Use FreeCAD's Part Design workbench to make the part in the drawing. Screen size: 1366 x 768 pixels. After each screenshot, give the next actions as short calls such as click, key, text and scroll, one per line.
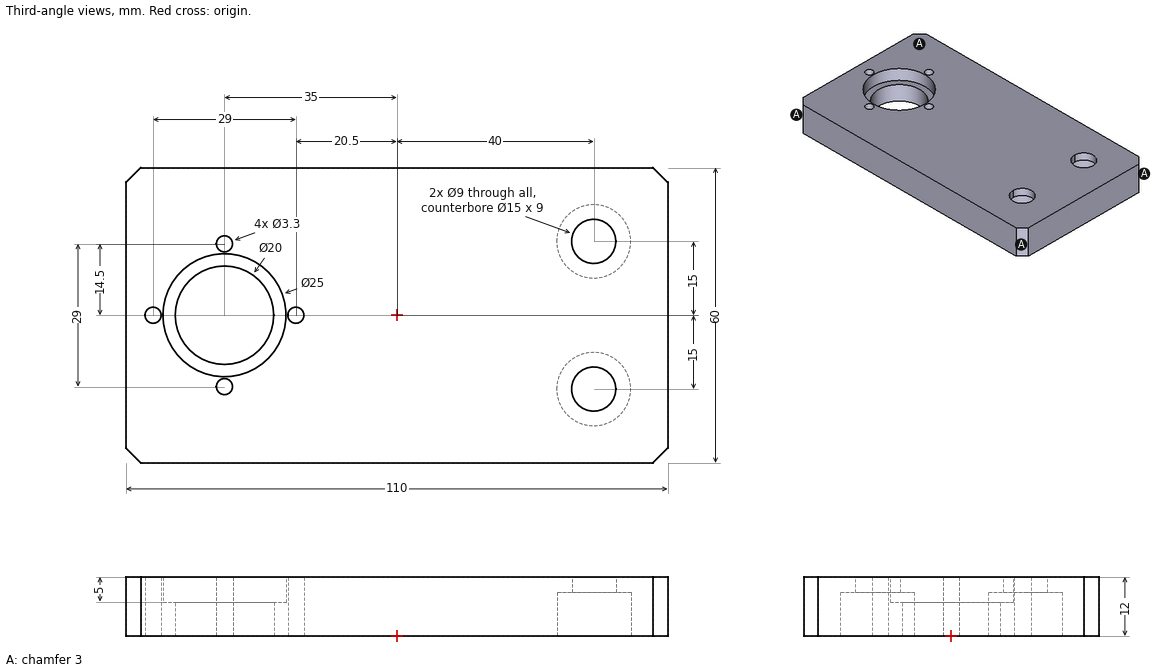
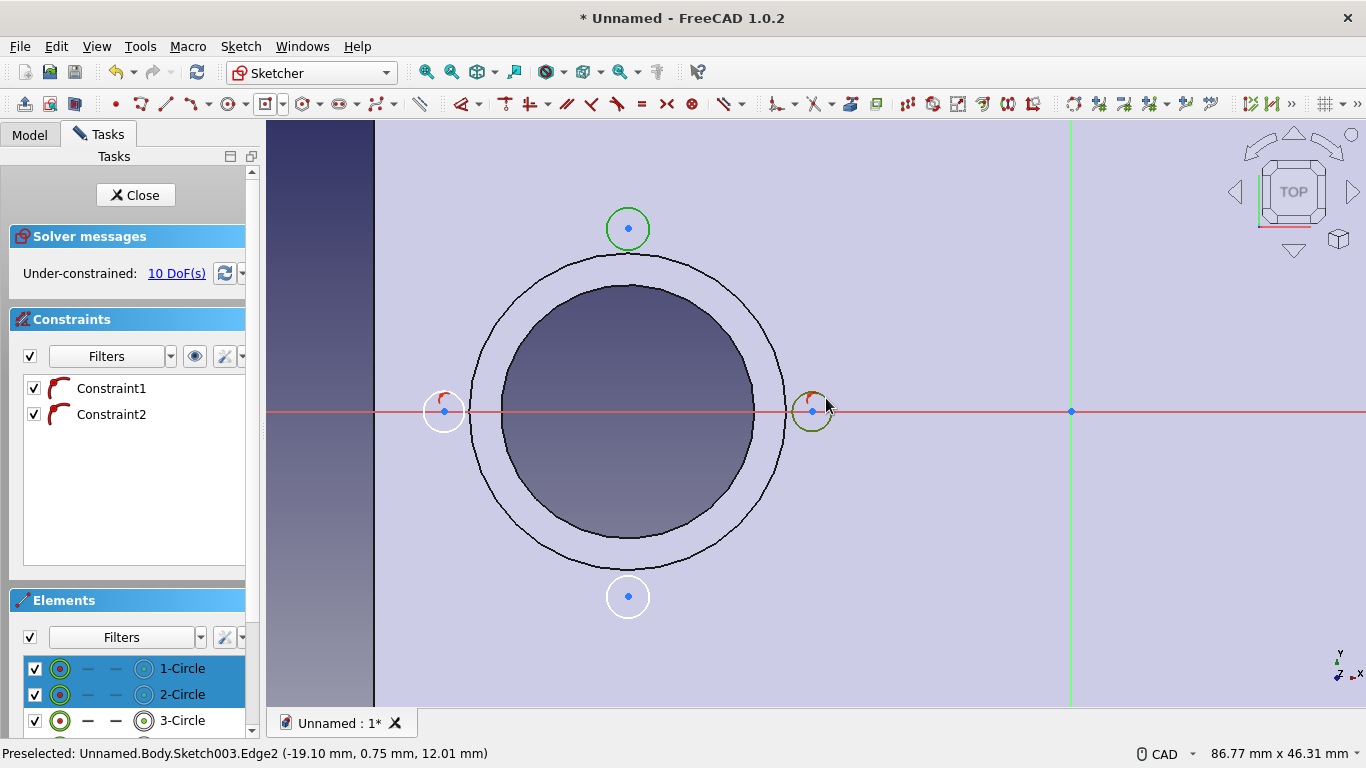
click(458, 397)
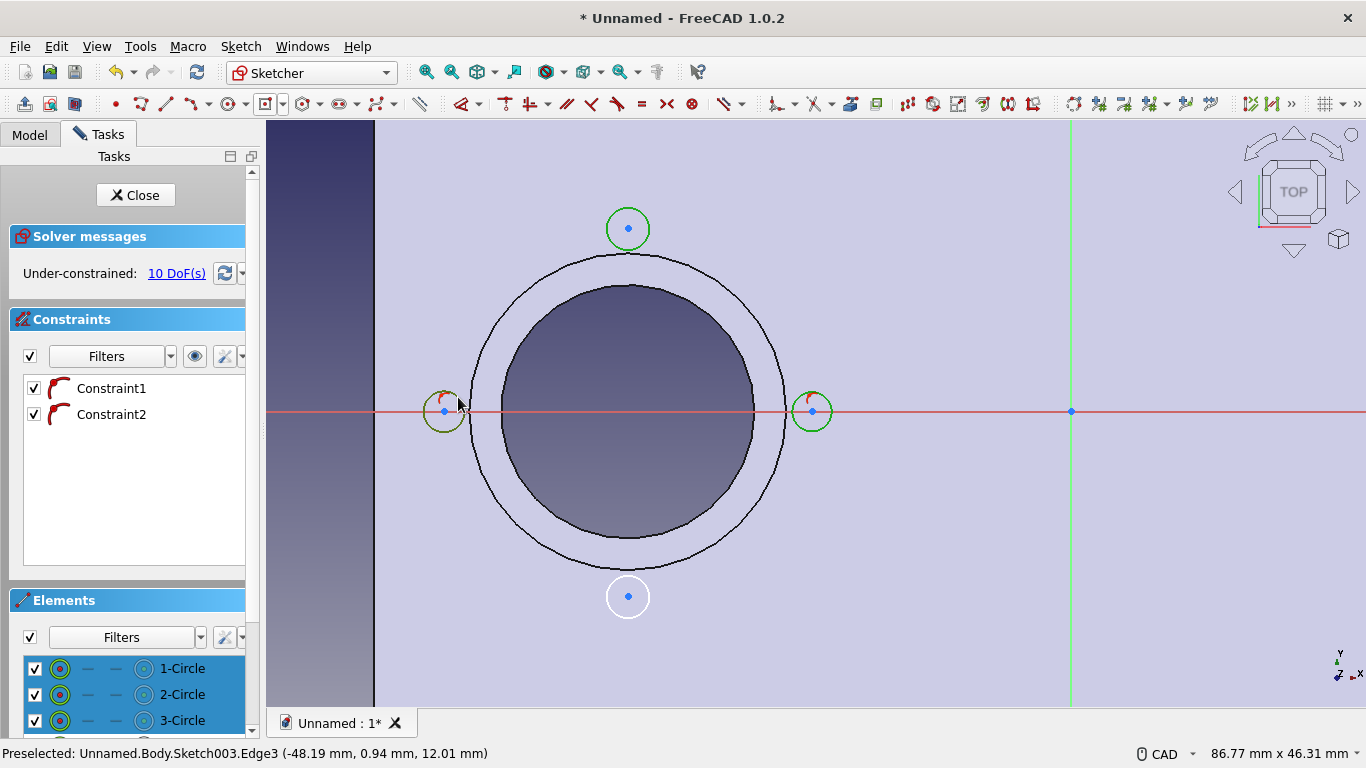
click(643, 582)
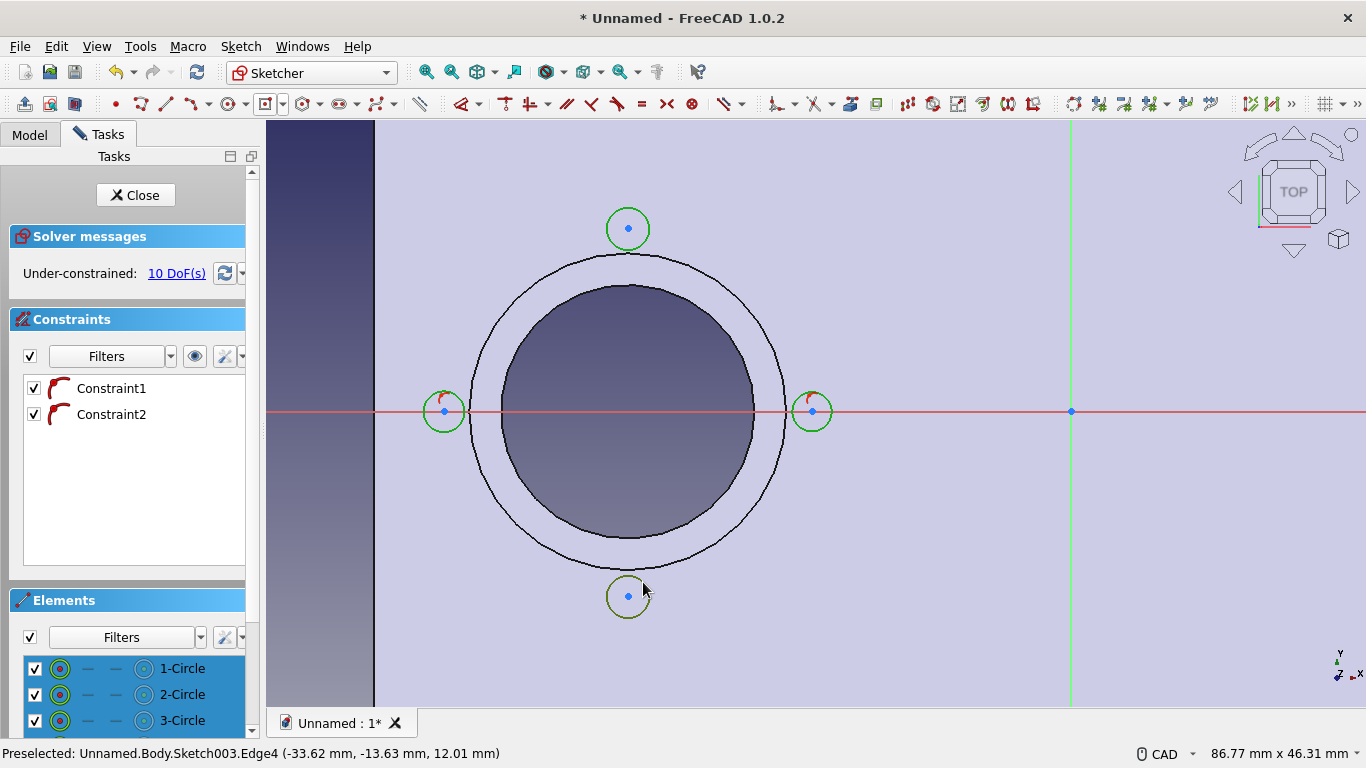
click(642, 104)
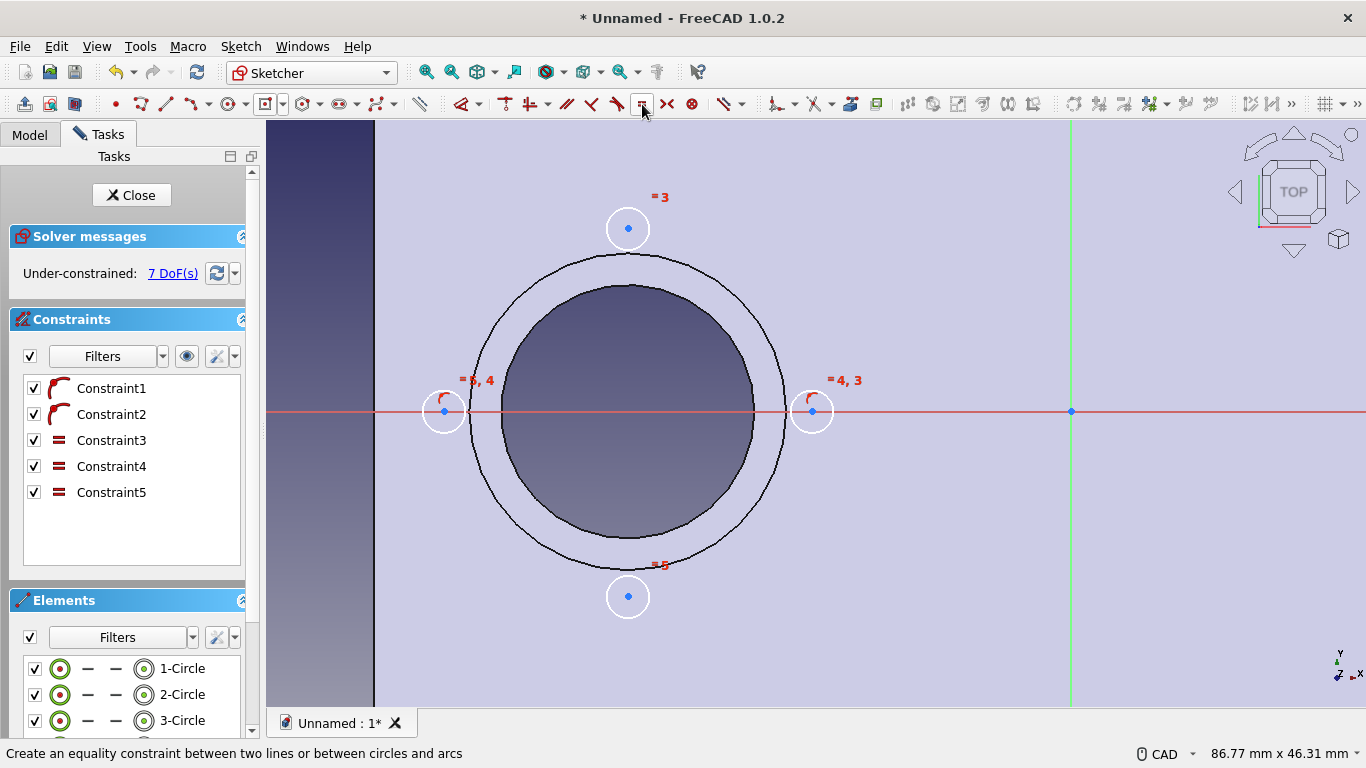
click(628, 229)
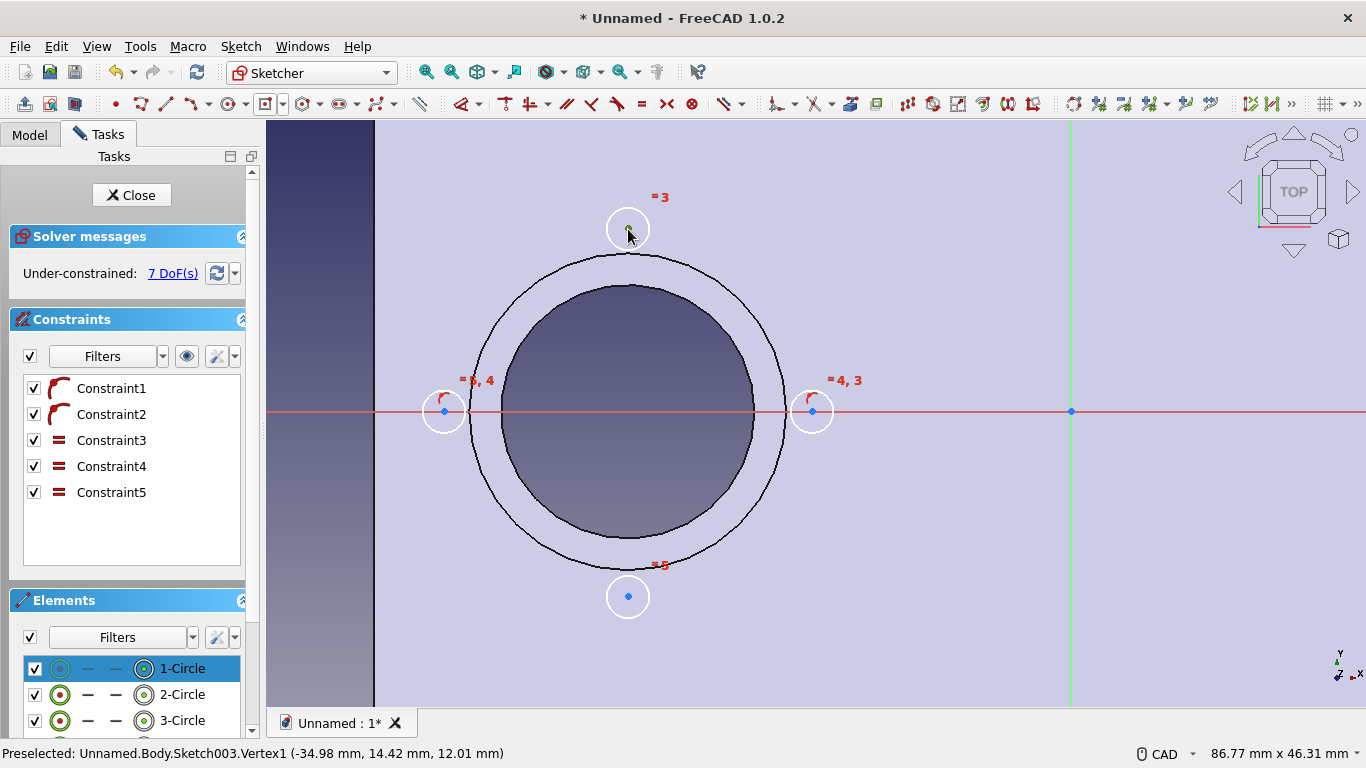
click(628, 597)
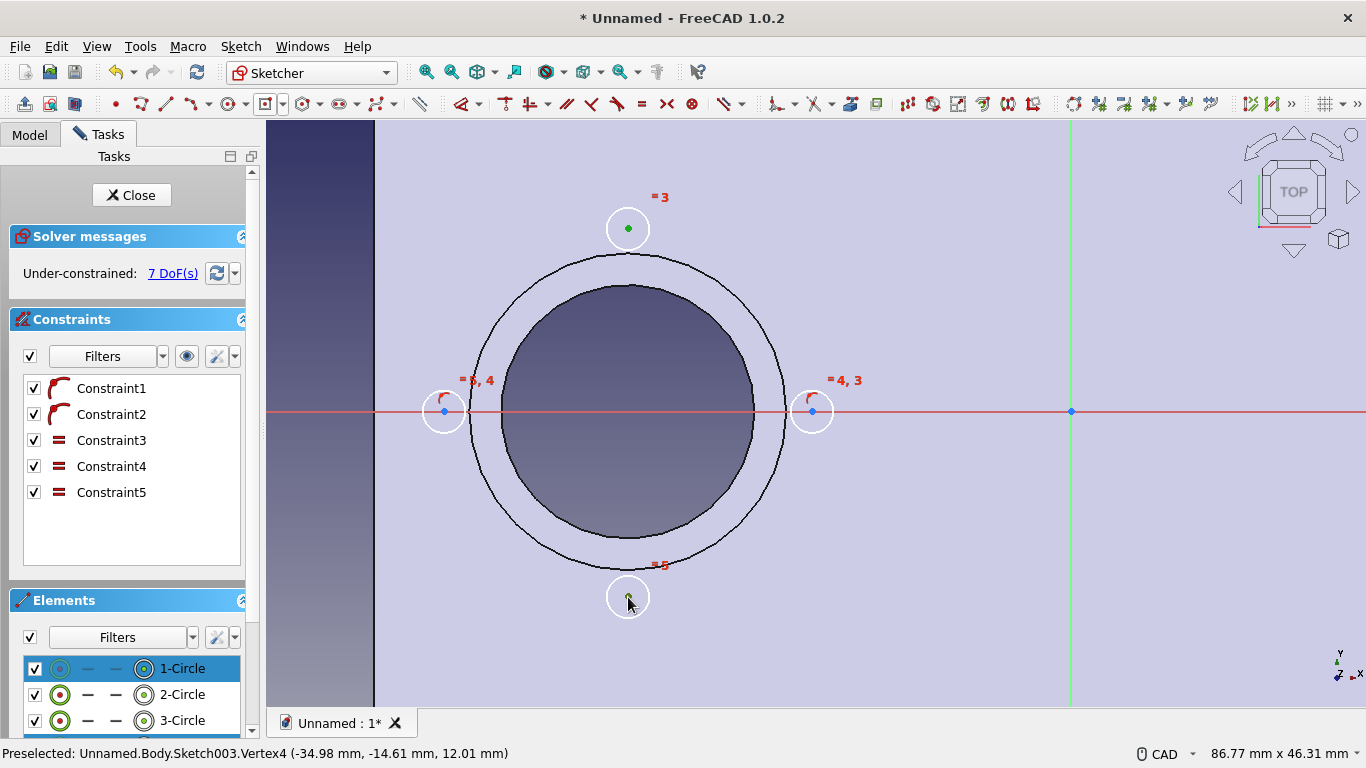
key(v)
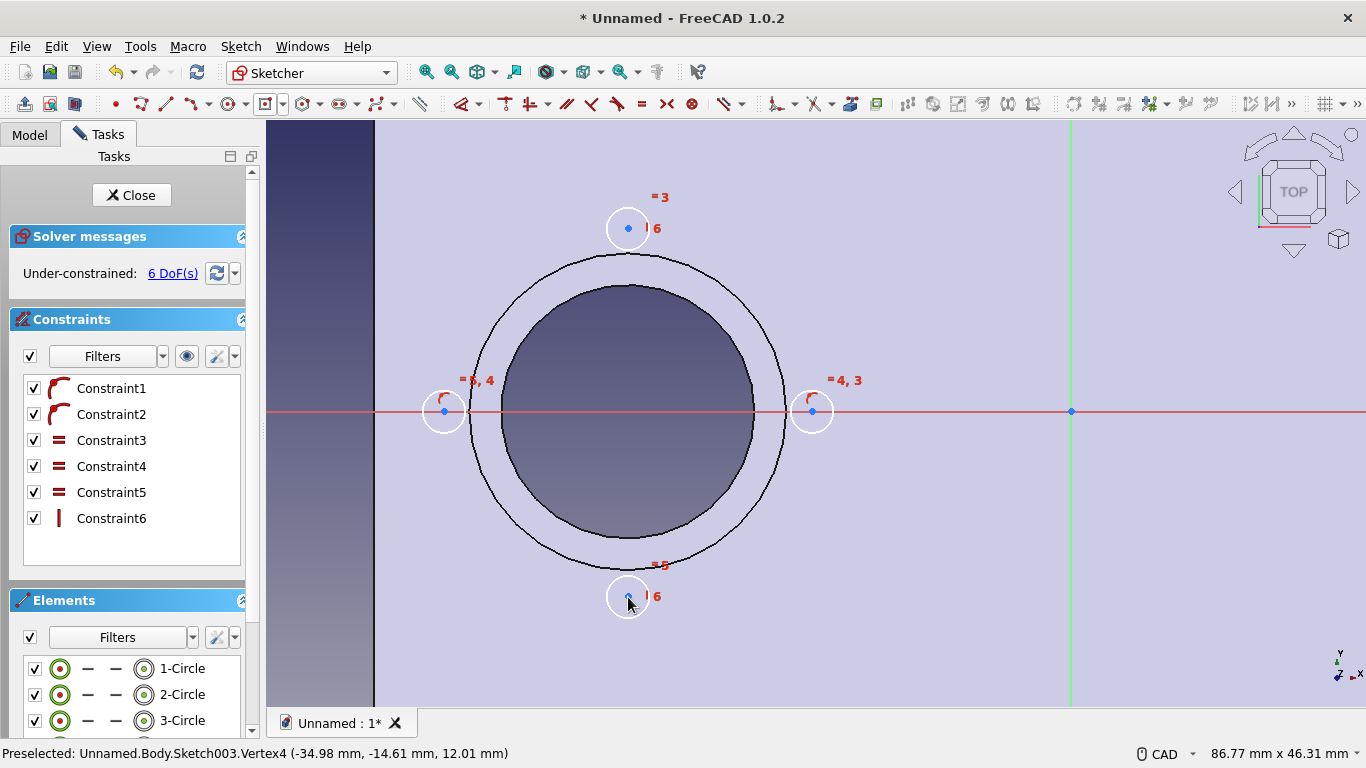
key(d)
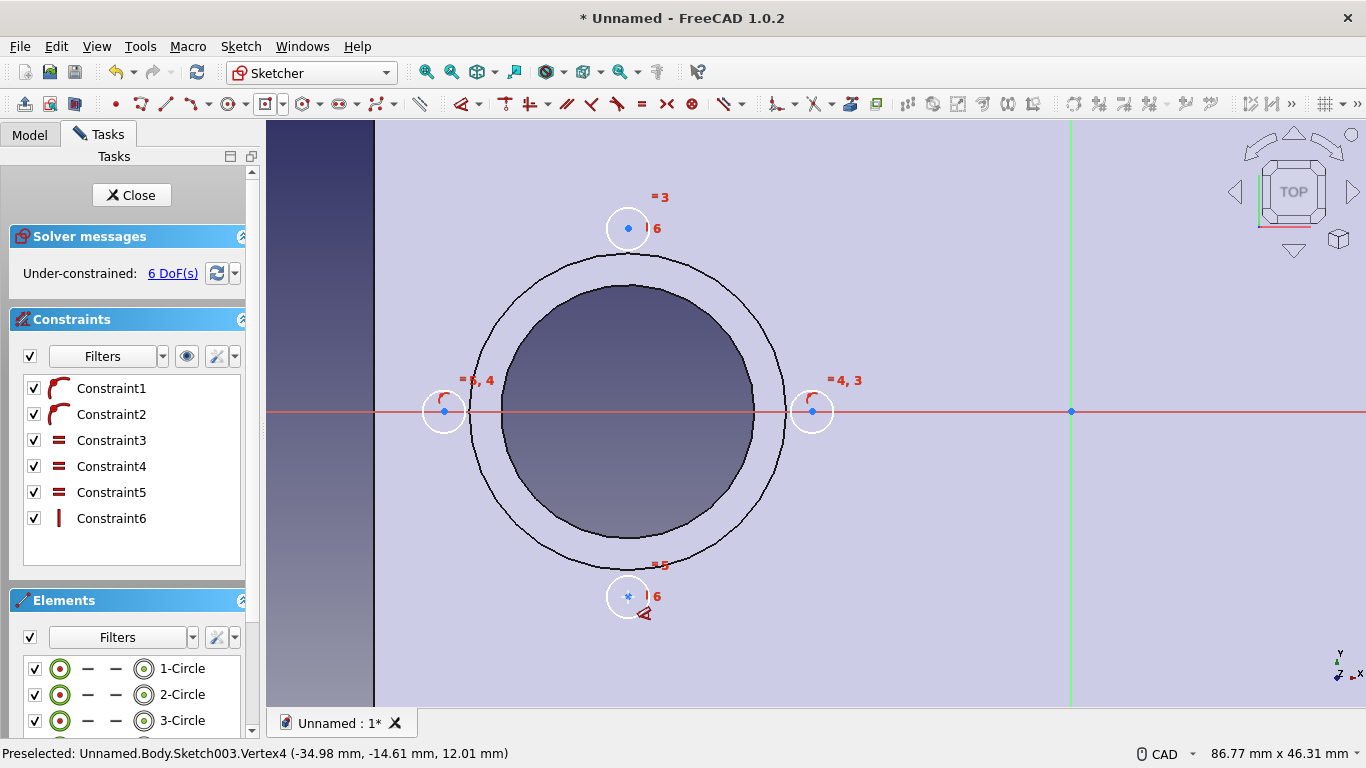
click(643, 214)
click(666, 191)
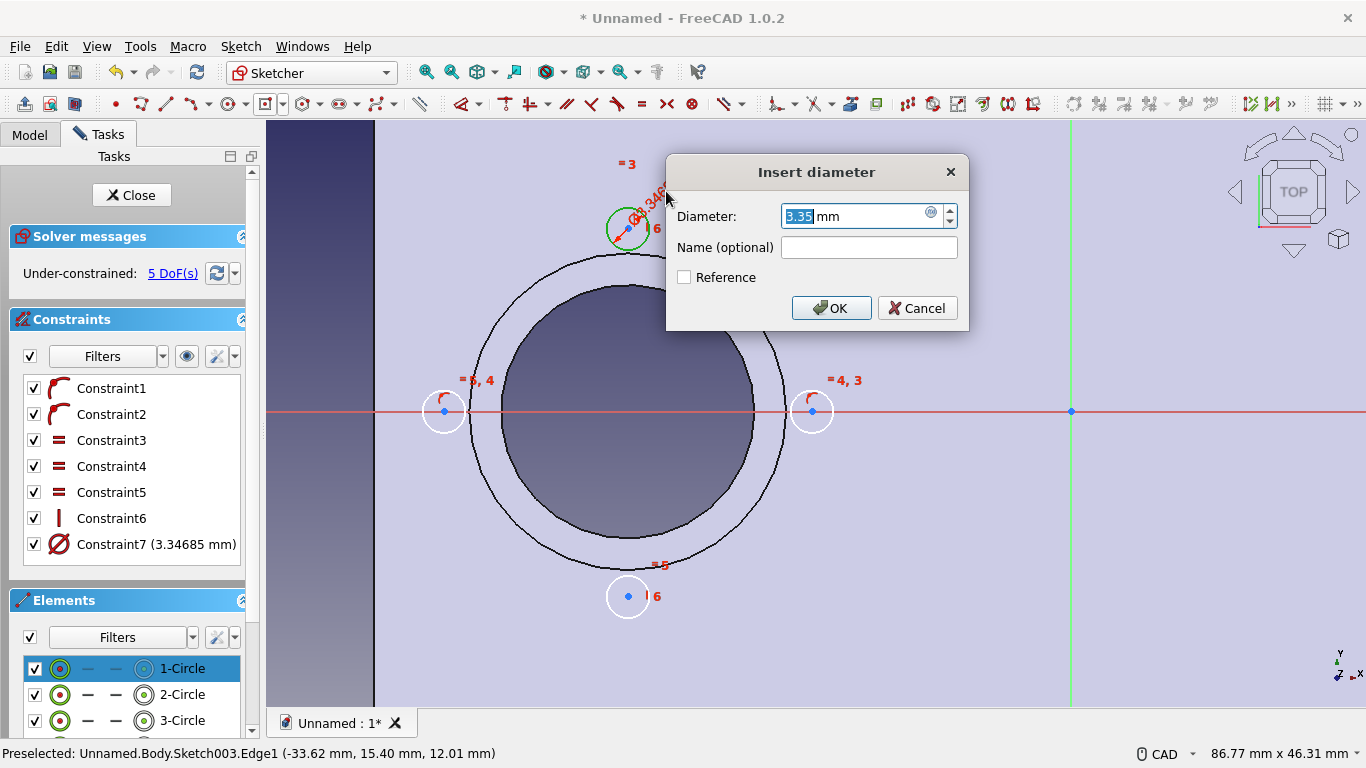
text(3.3)
key(Return)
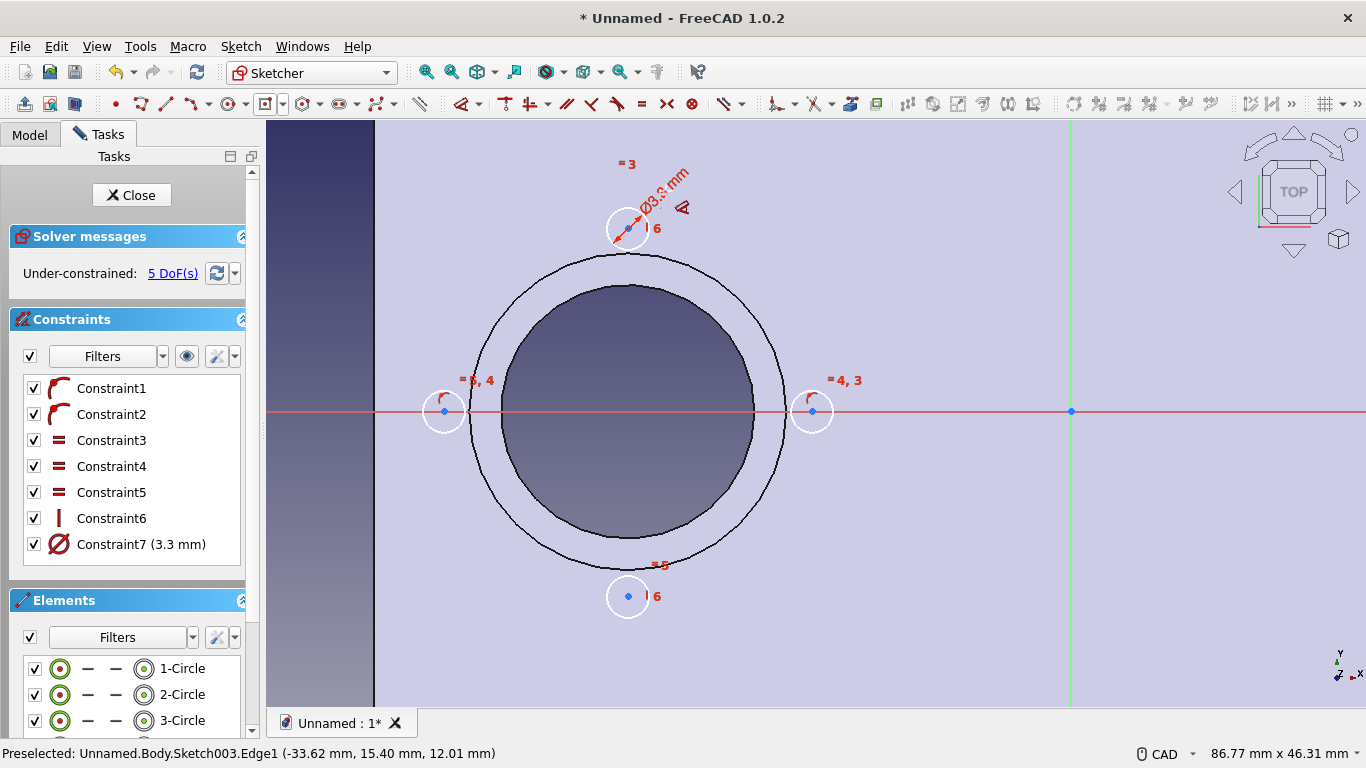
click(628, 229)
click(850, 195)